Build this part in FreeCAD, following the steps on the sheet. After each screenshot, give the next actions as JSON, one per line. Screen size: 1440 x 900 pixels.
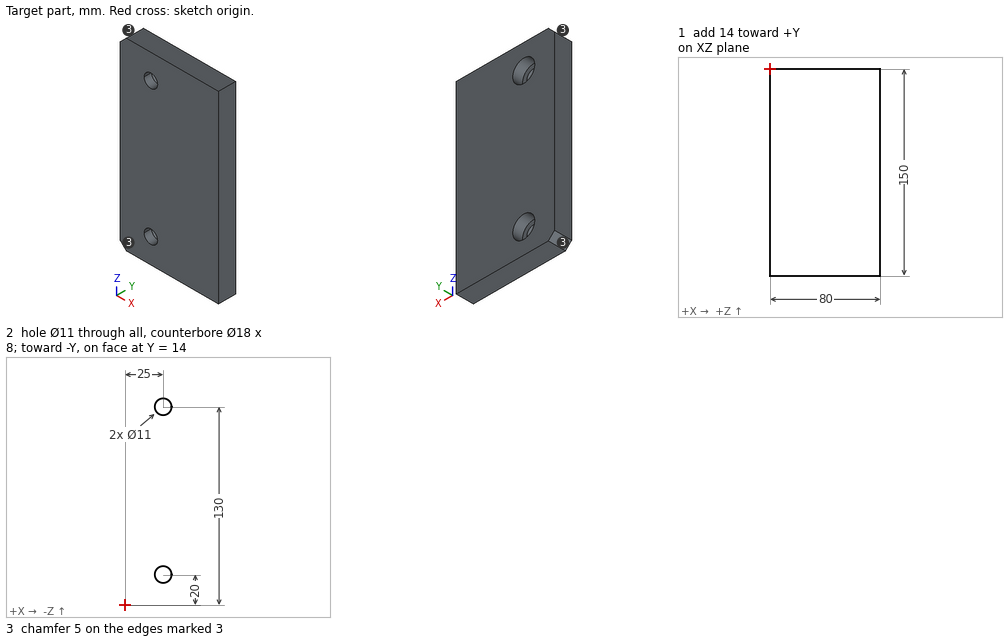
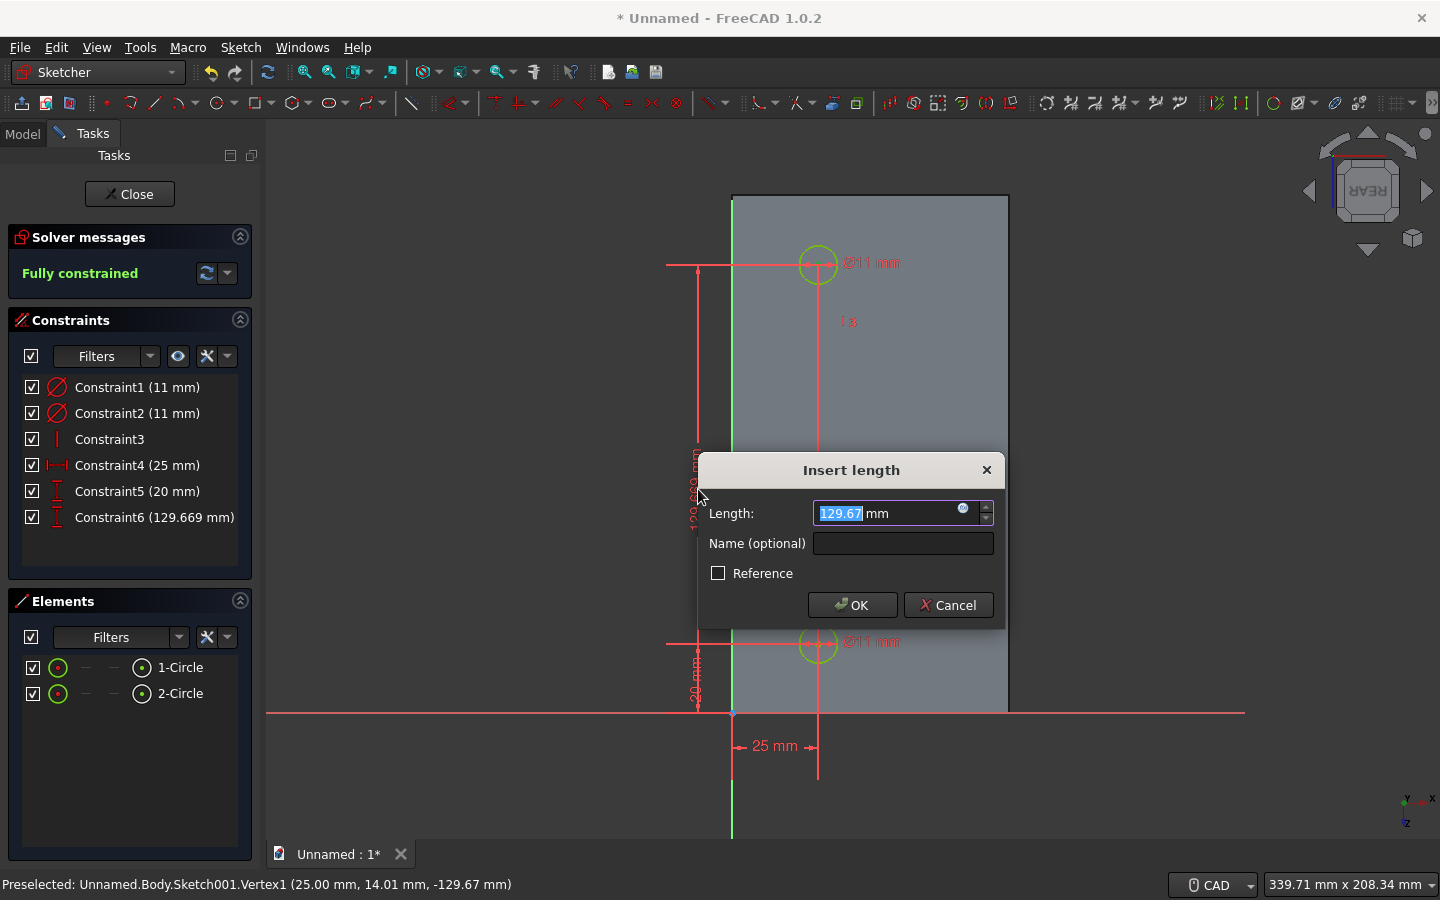
{"action": "type", "text": "130"}
{"action": "key", "text": "Return"}
{"action": "key", "text": "Escape"}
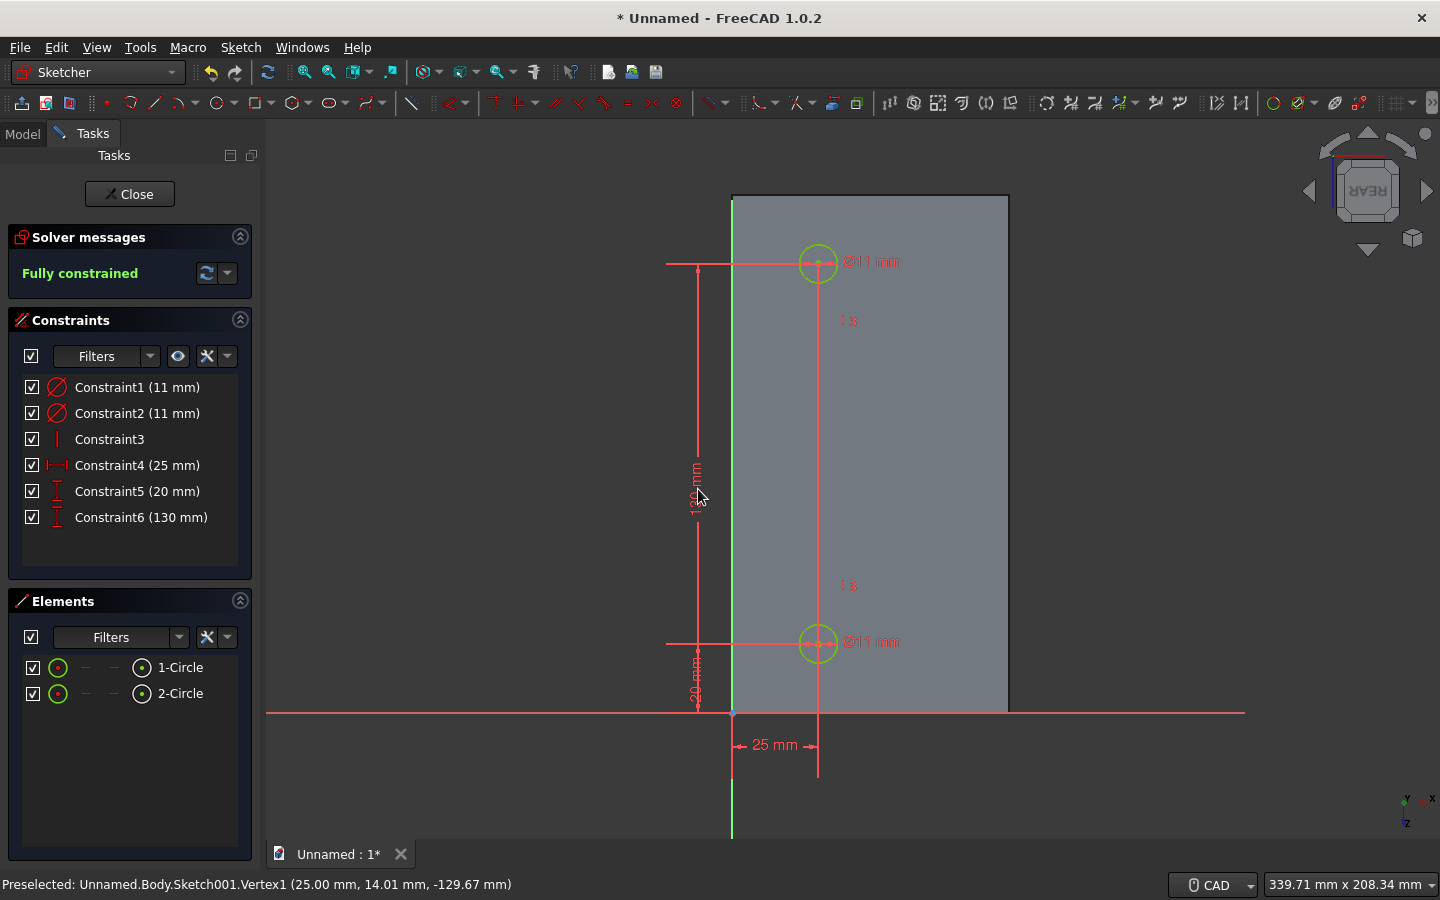
{"action": "left_click", "coordinate": [130, 194]}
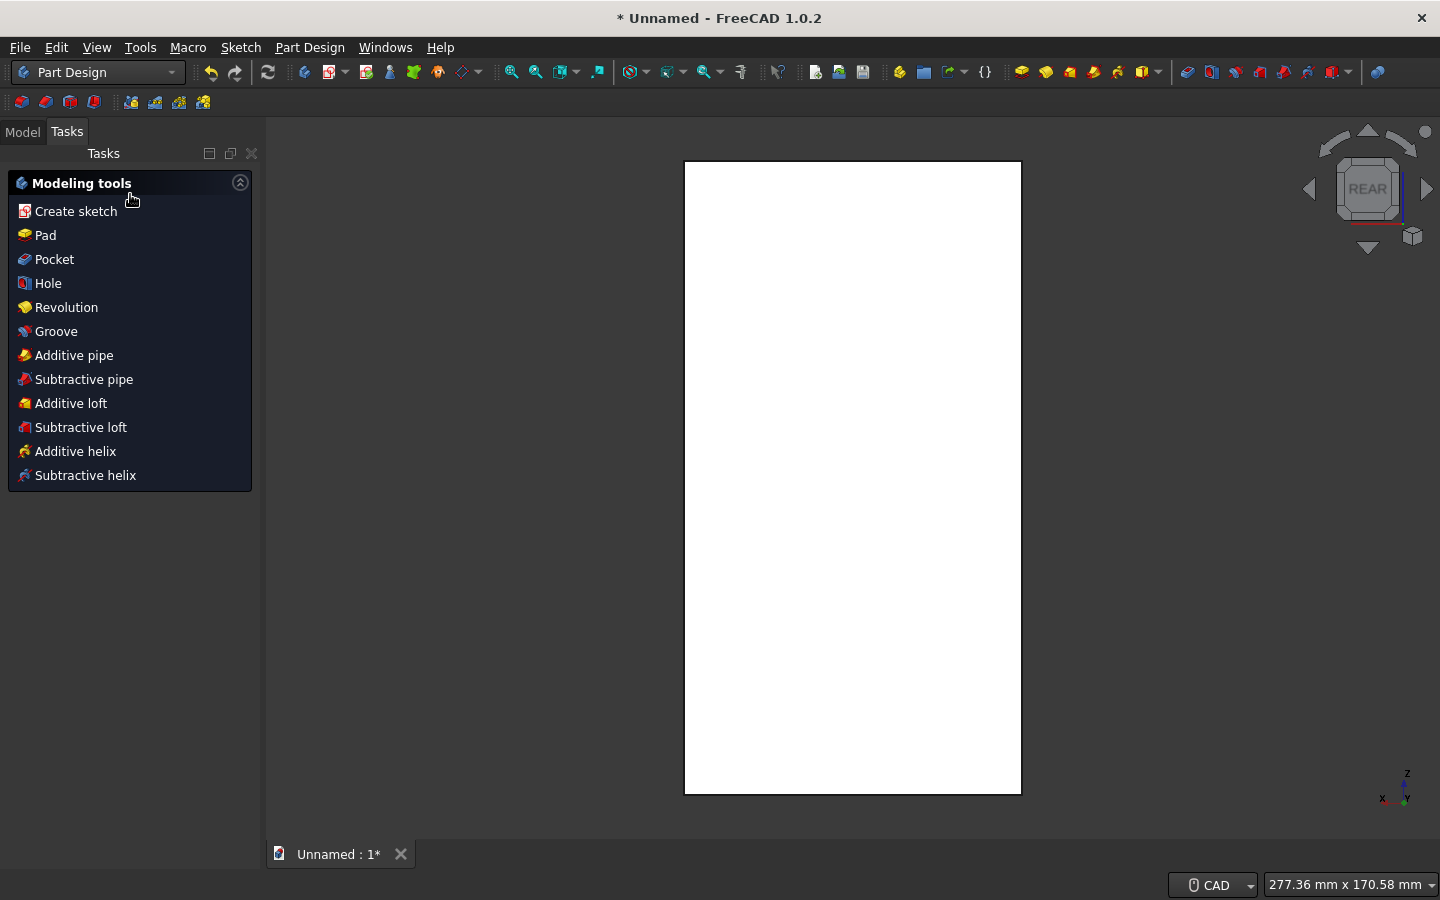
{"action": "left_click", "coordinate": [1212, 72]}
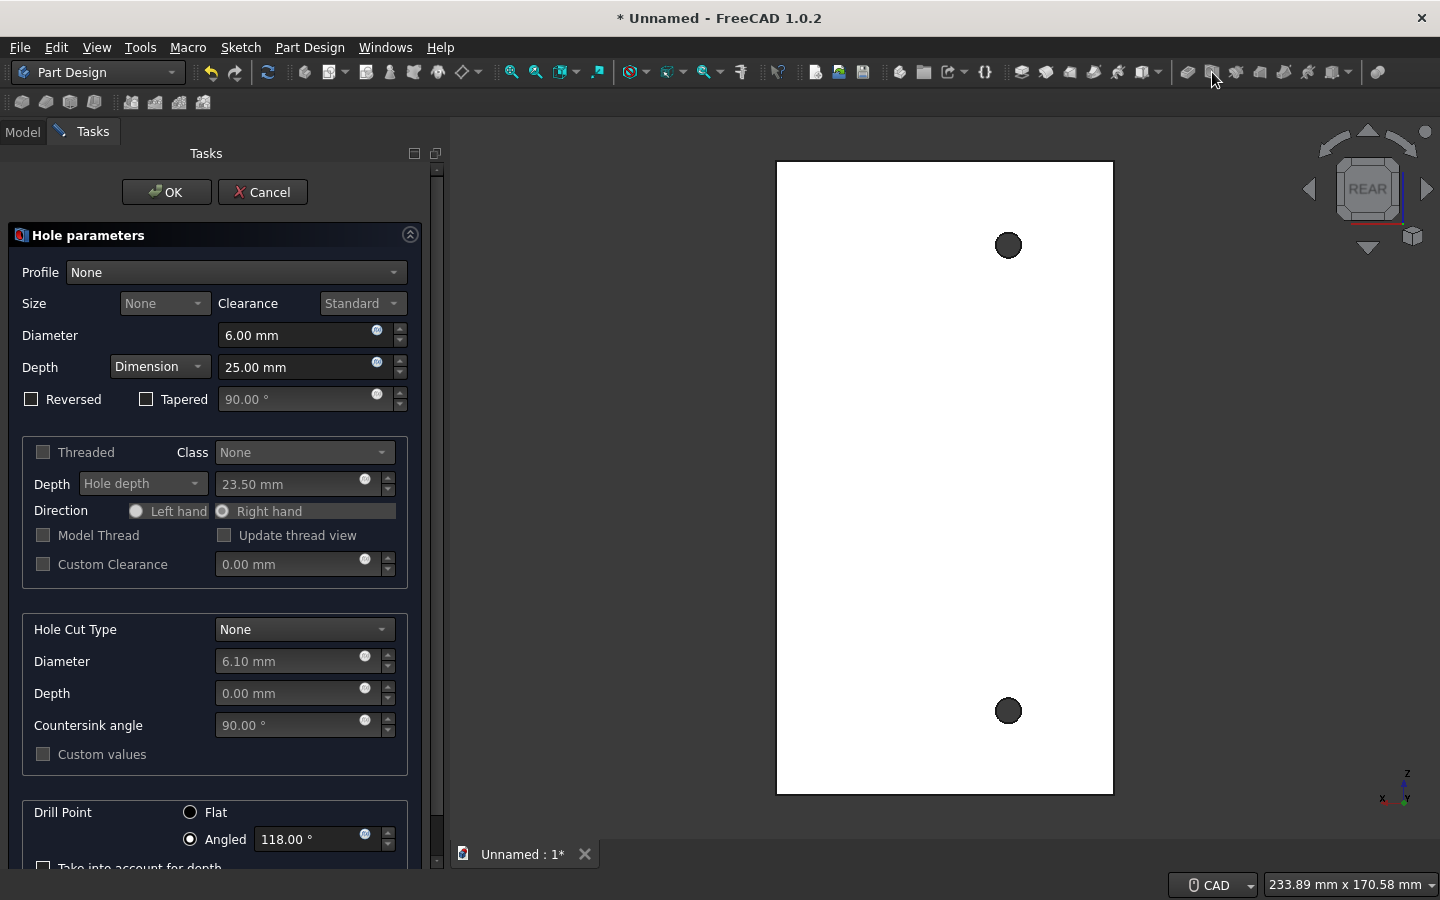
{"action": "triple_click", "coordinate": [305, 335]}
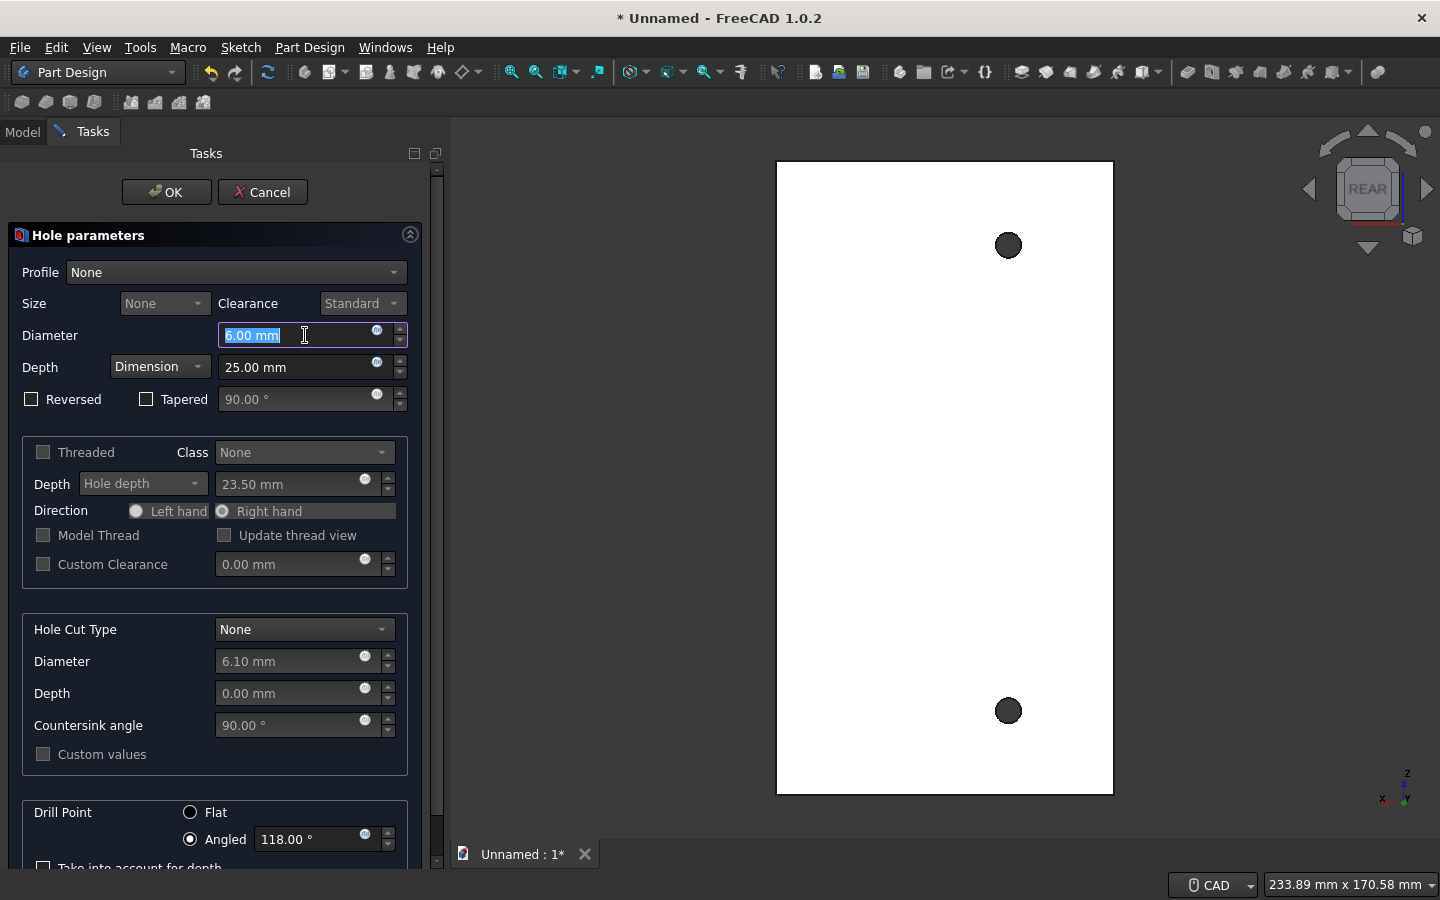
{"action": "type", "text": "11"}
{"action": "key", "text": "Tab"}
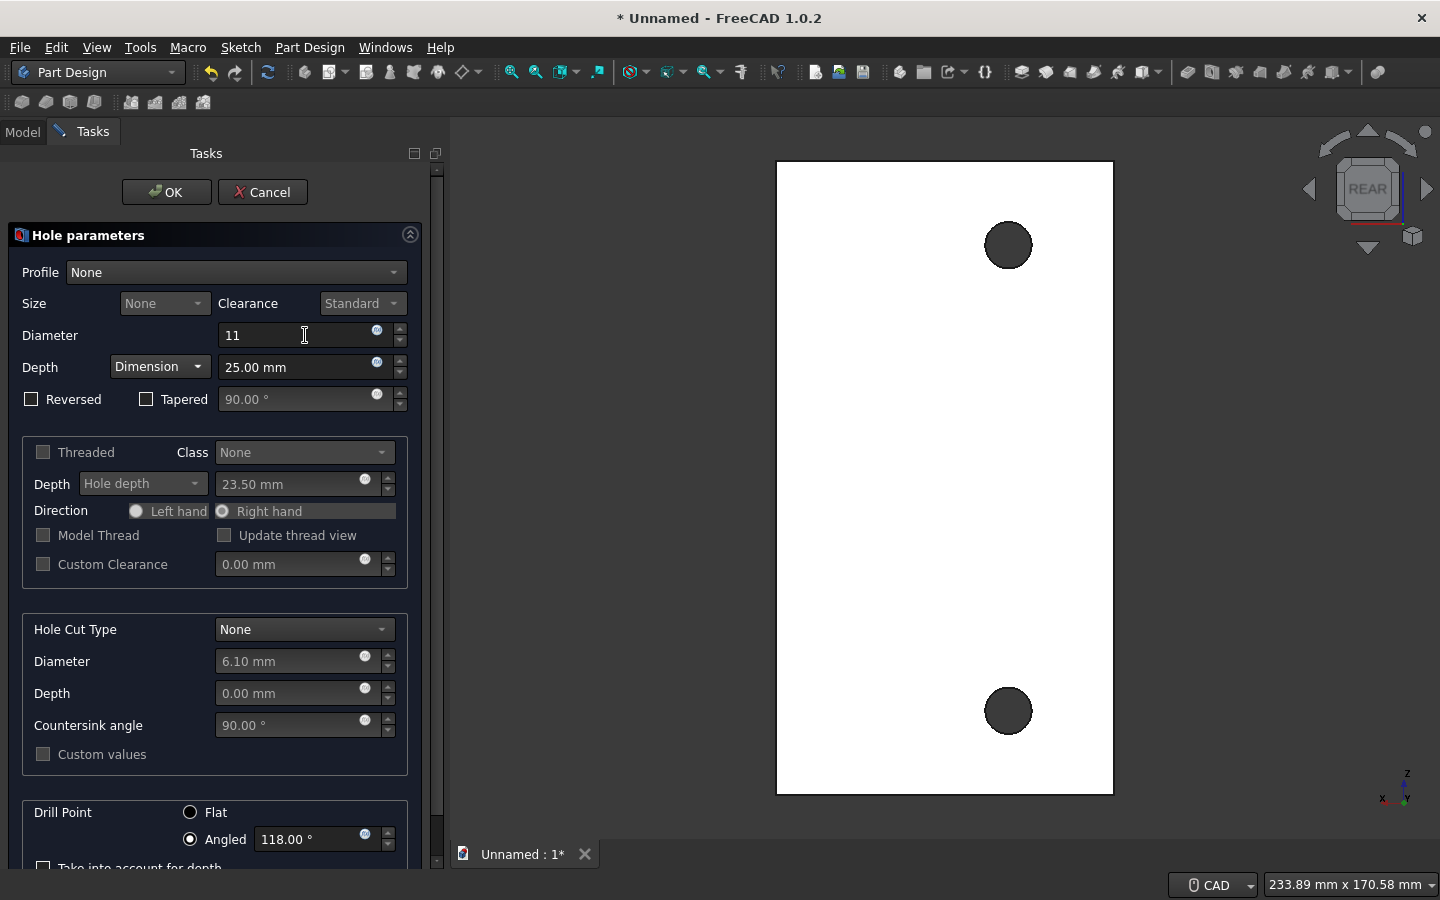
{"action": "left_click", "coordinate": [161, 366]}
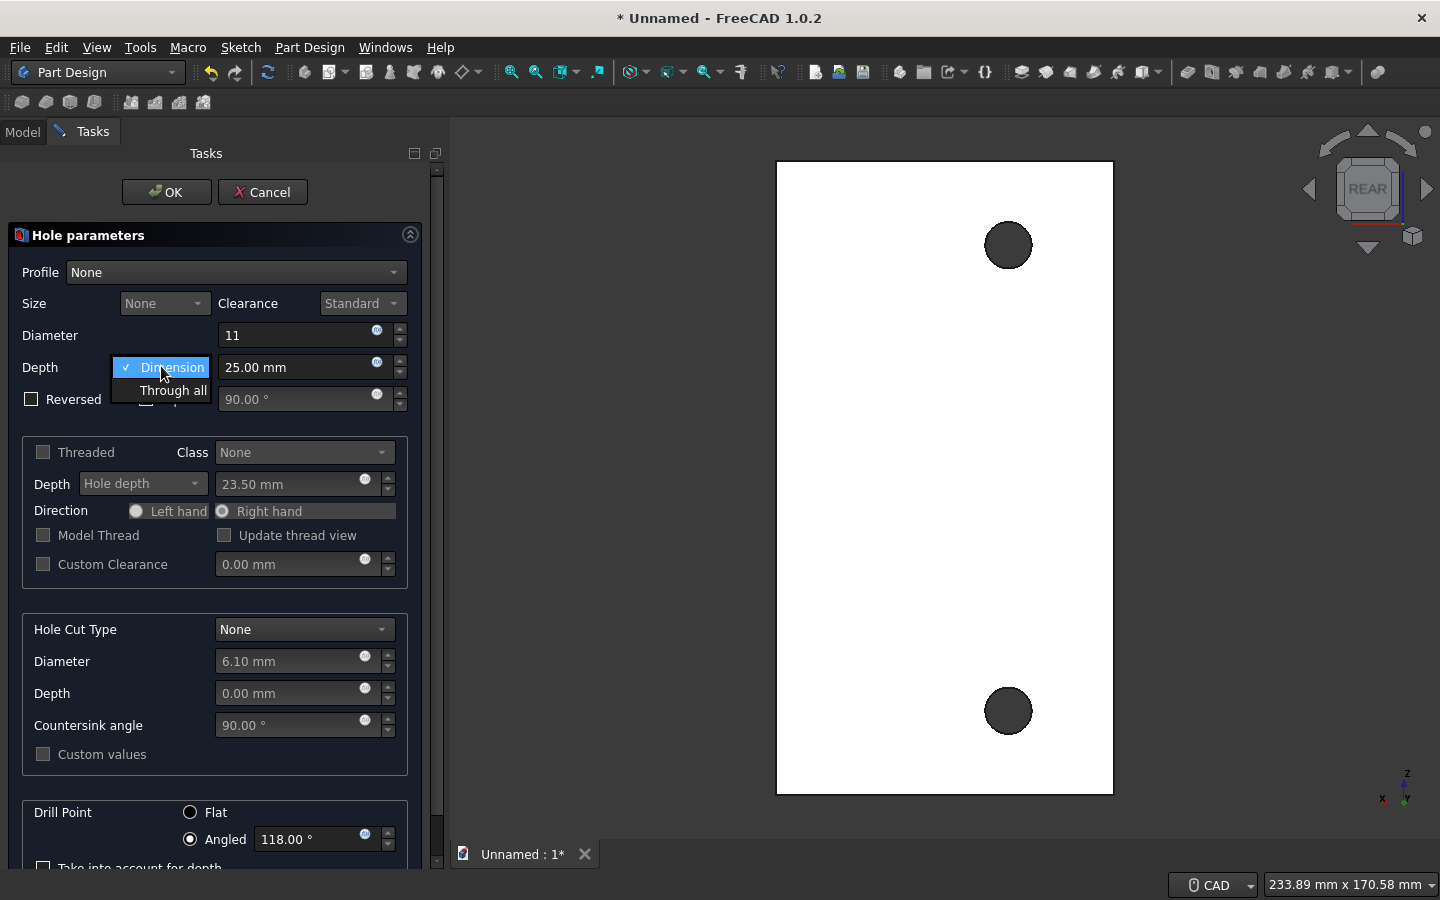
{"action": "left_click", "coordinate": [160, 390]}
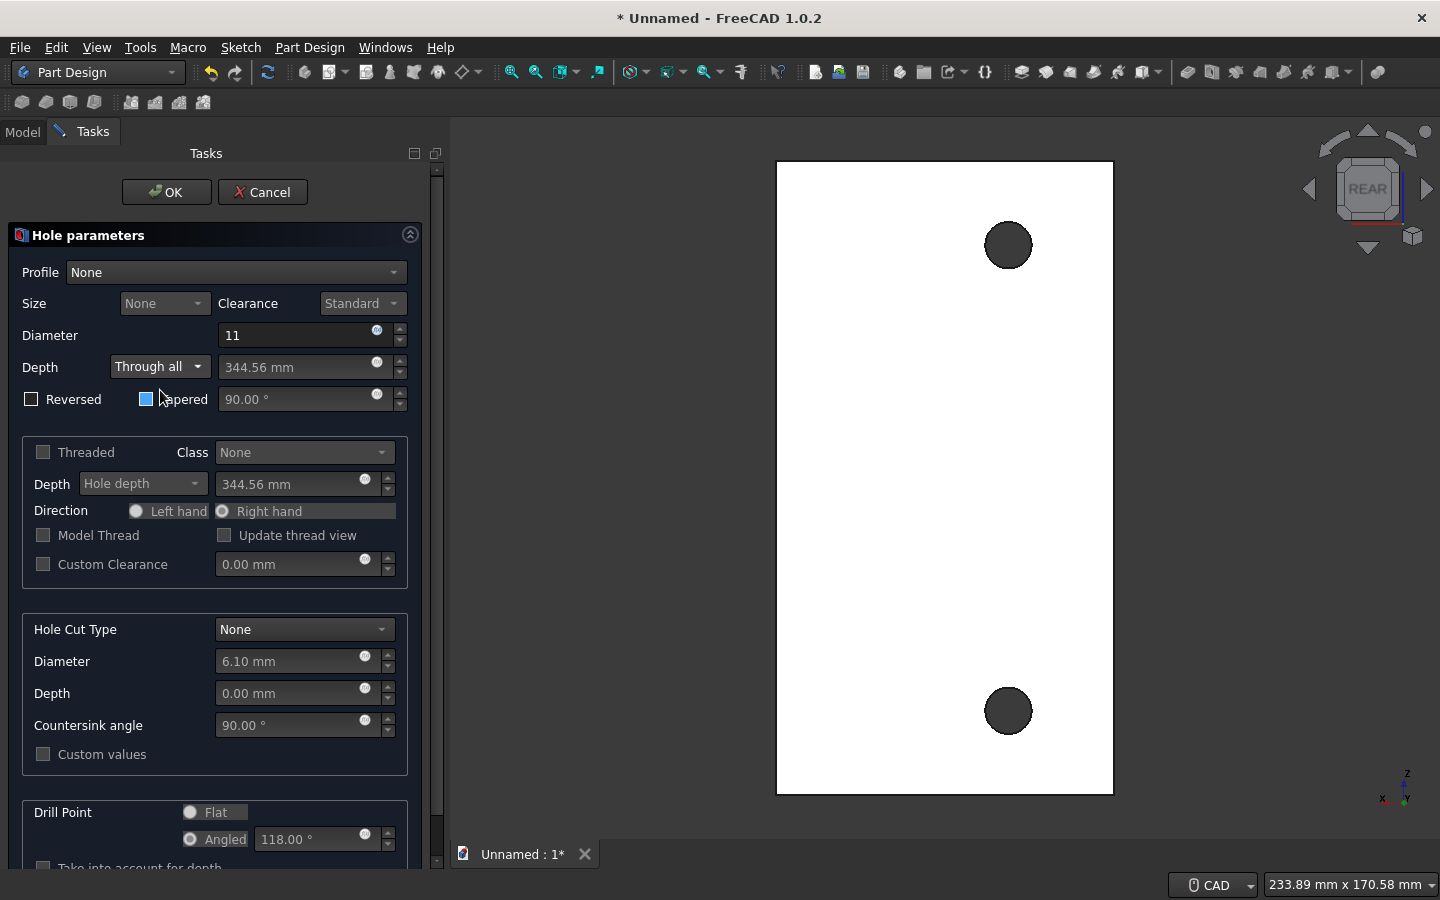
{"action": "left_click", "coordinate": [306, 630]}